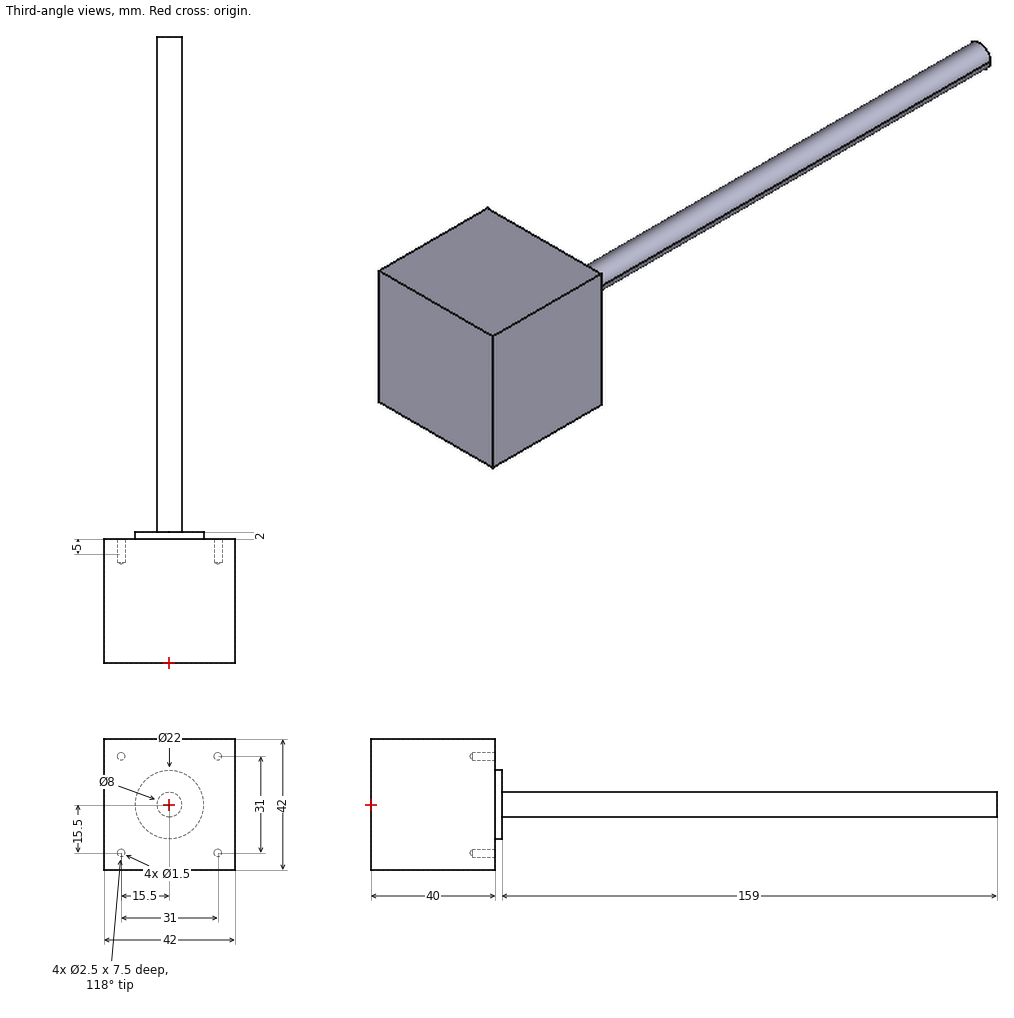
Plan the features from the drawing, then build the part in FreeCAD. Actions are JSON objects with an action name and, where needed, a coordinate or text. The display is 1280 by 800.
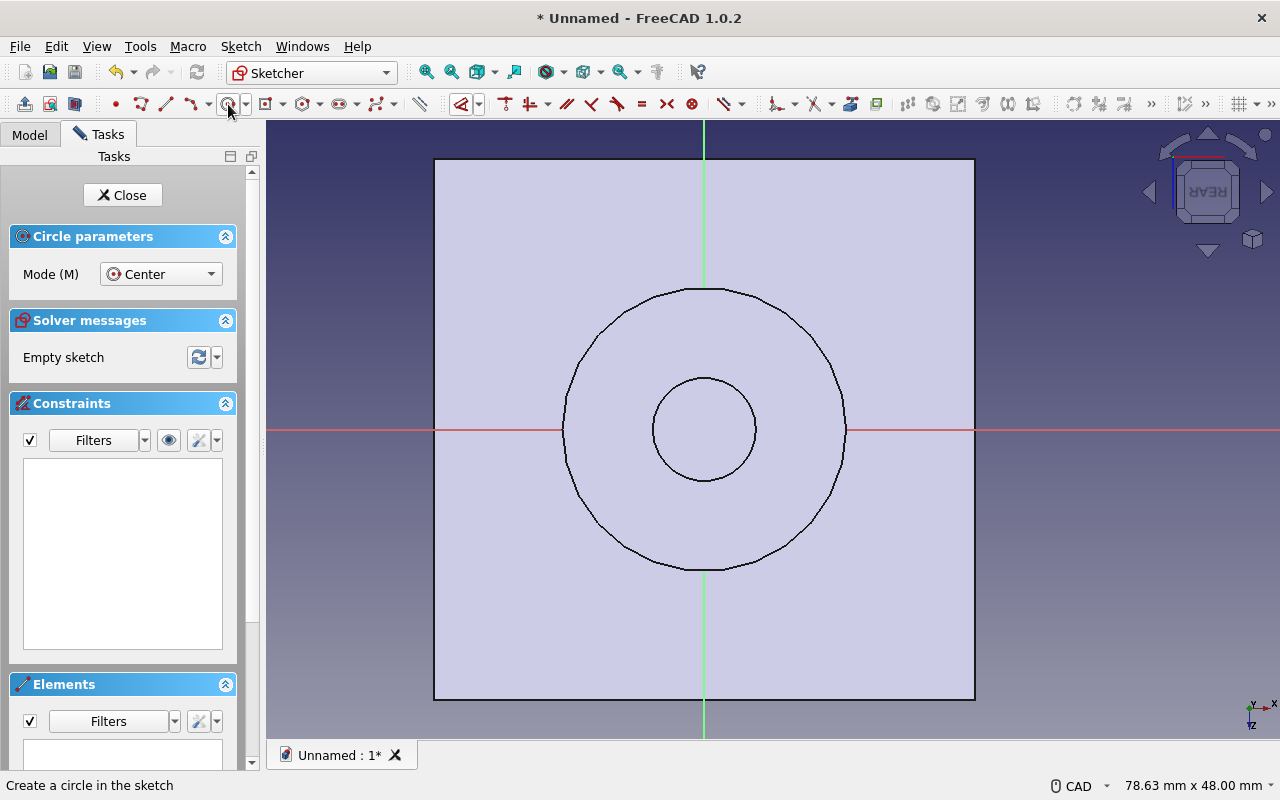
{"action": "scroll", "coordinate": [504, 230], "scroll_direction": "up", "scroll_amount": 5}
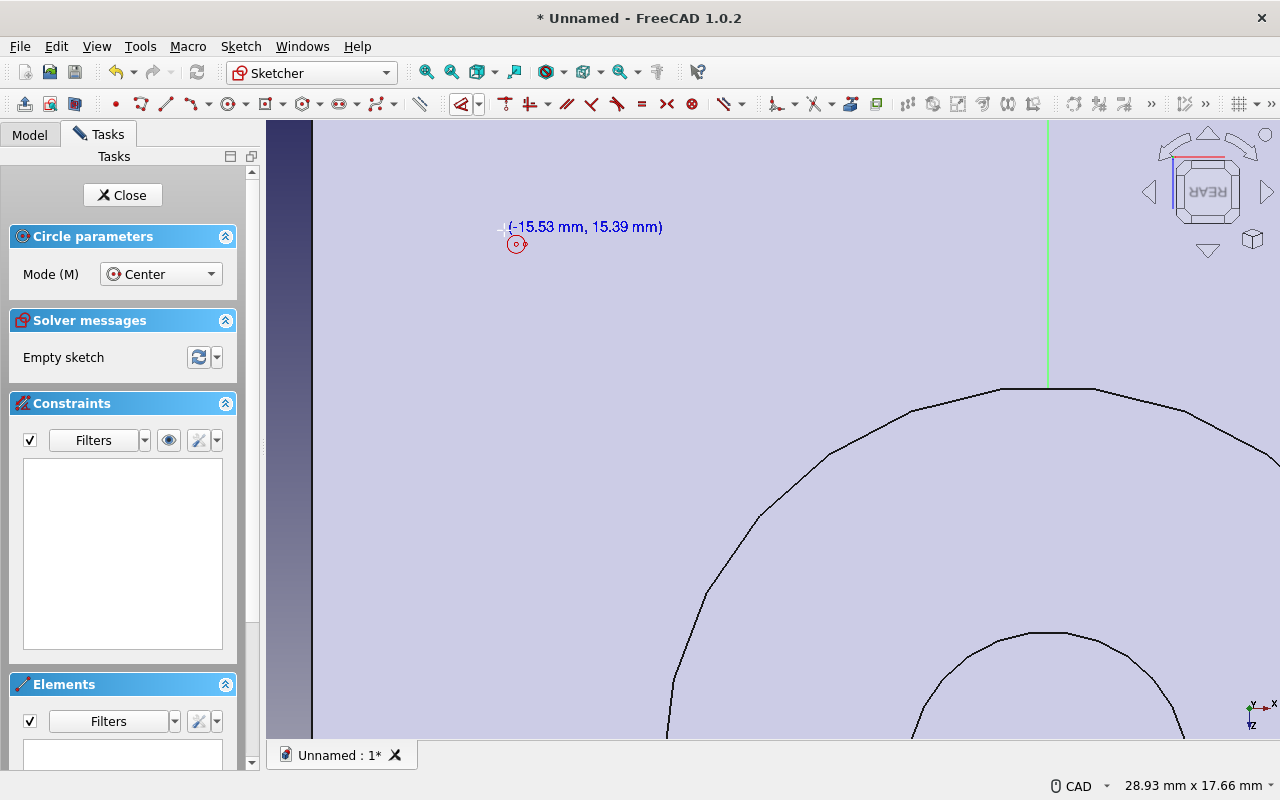
{"action": "left_click", "coordinate": [505, 229]}
{"action": "left_click", "coordinate": [523, 210]}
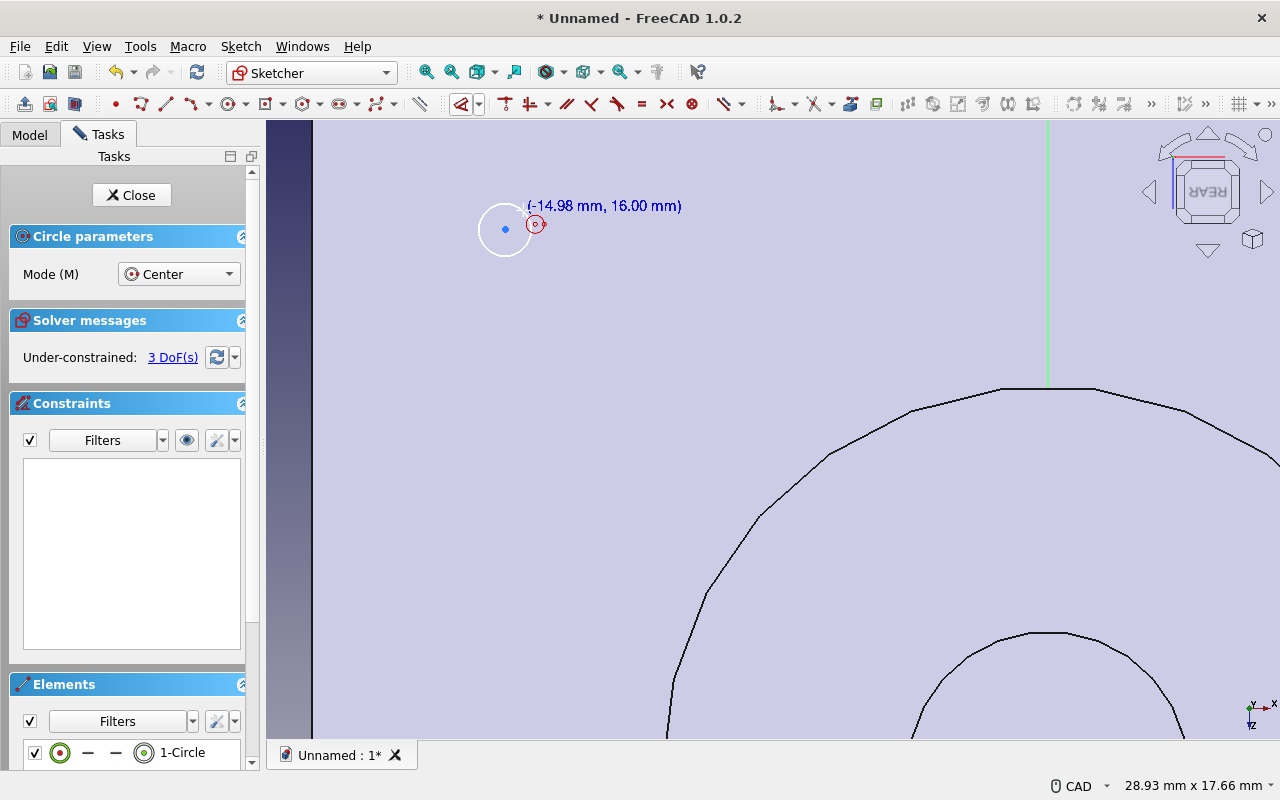
{"action": "scroll", "coordinate": [505, 230], "scroll_direction": "down", "scroll_amount": 5}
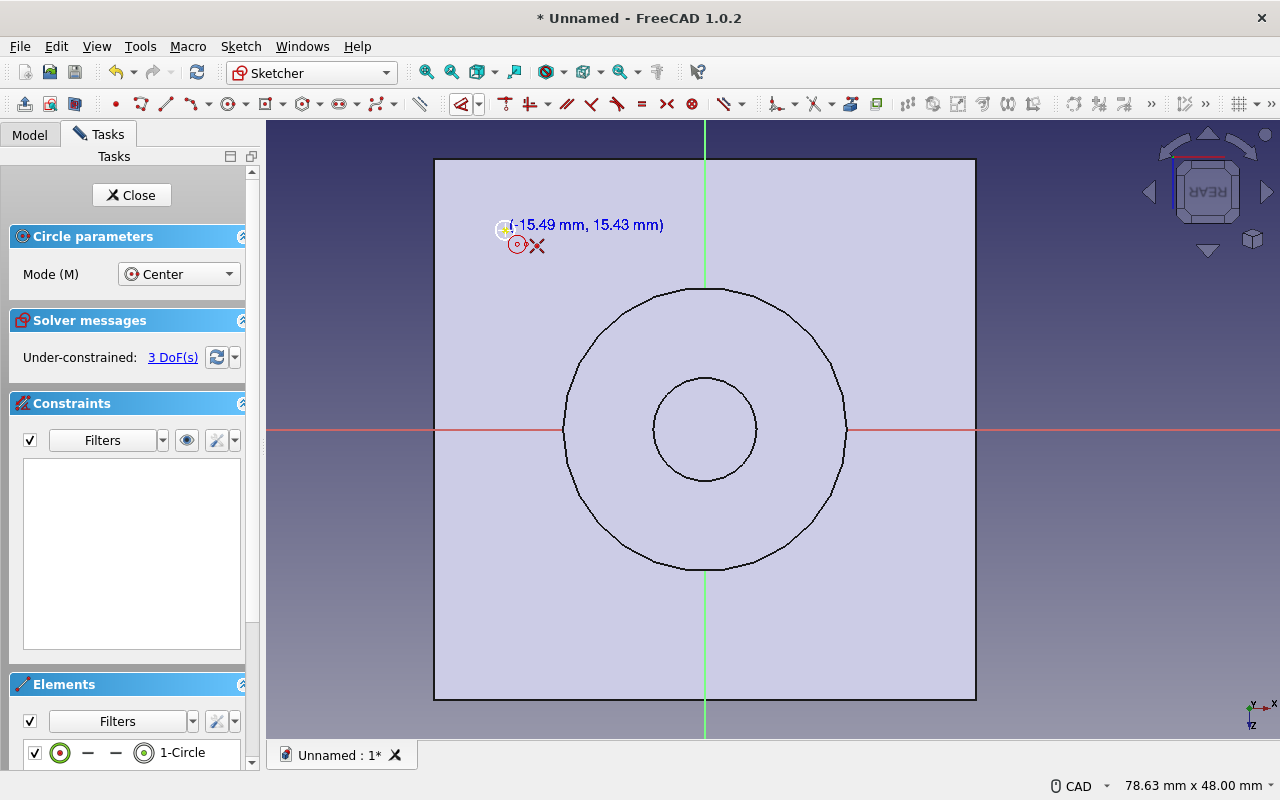
{"action": "scroll", "coordinate": [905, 230], "scroll_direction": "up", "scroll_amount": 5}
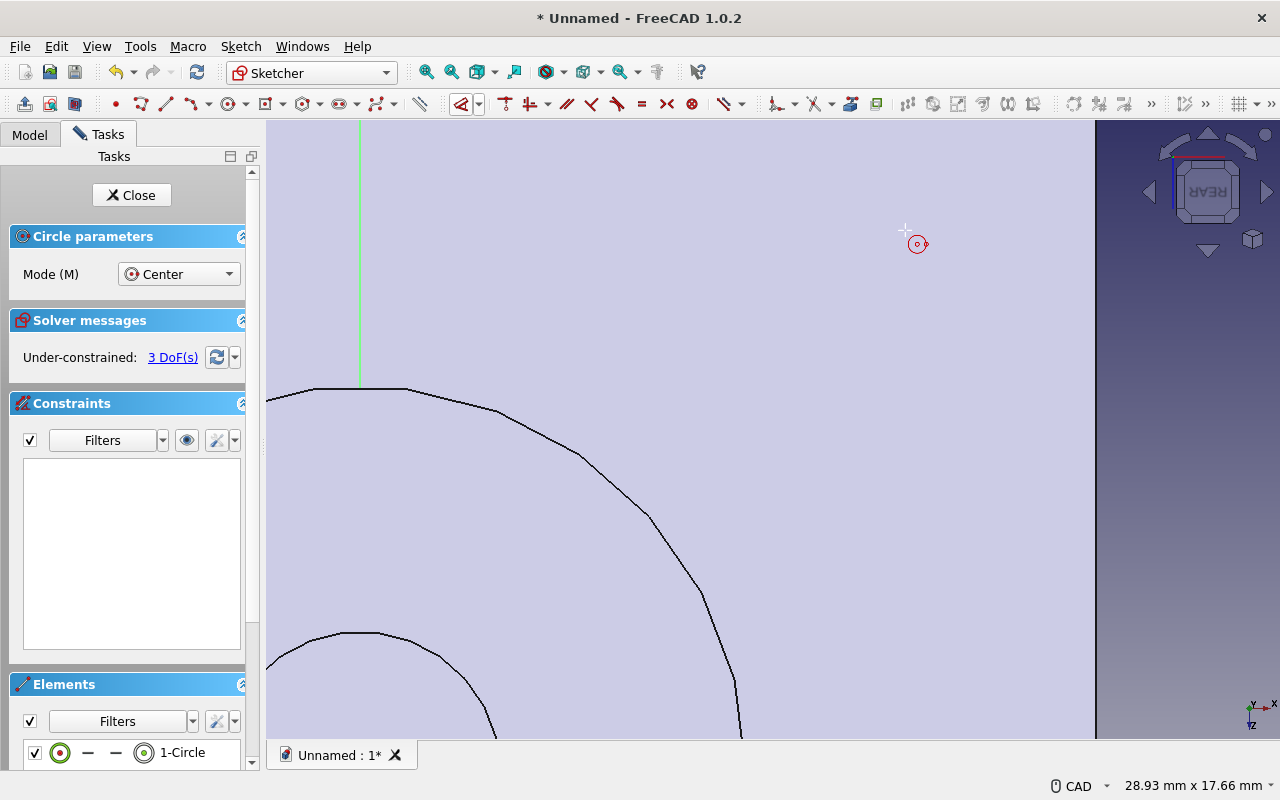
{"action": "left_click", "coordinate": [903, 229]}
{"action": "left_click", "coordinate": [922, 210]}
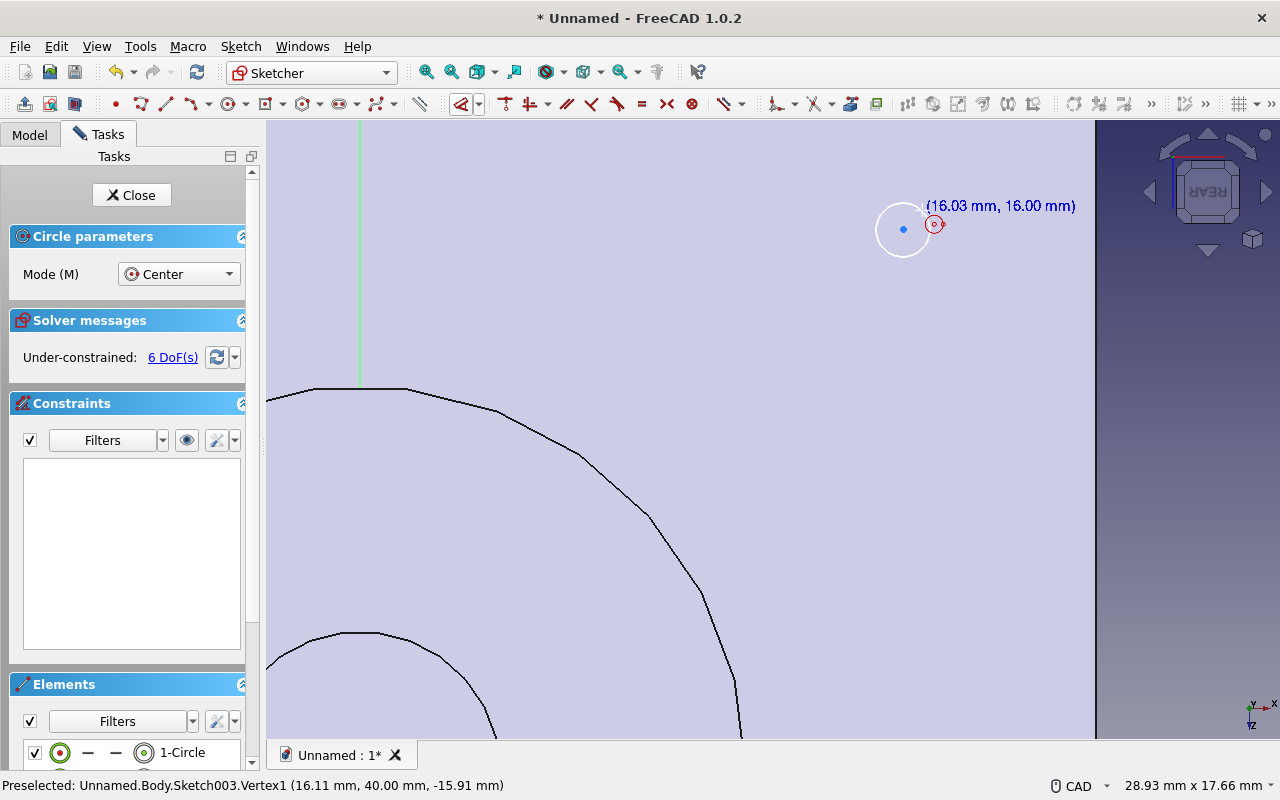
{"action": "scroll", "coordinate": [905, 230], "scroll_direction": "down", "scroll_amount": 5}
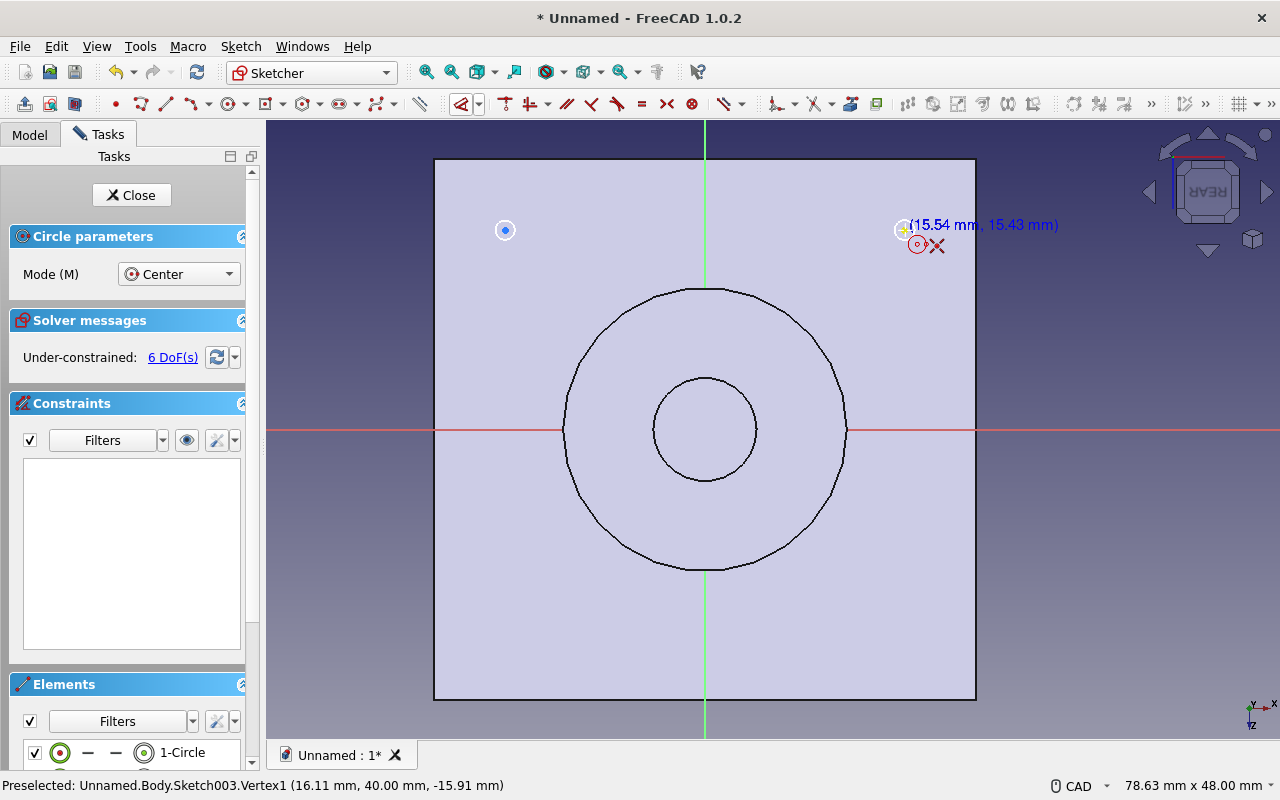
{"action": "scroll", "coordinate": [905, 629], "scroll_direction": "up", "scroll_amount": 5}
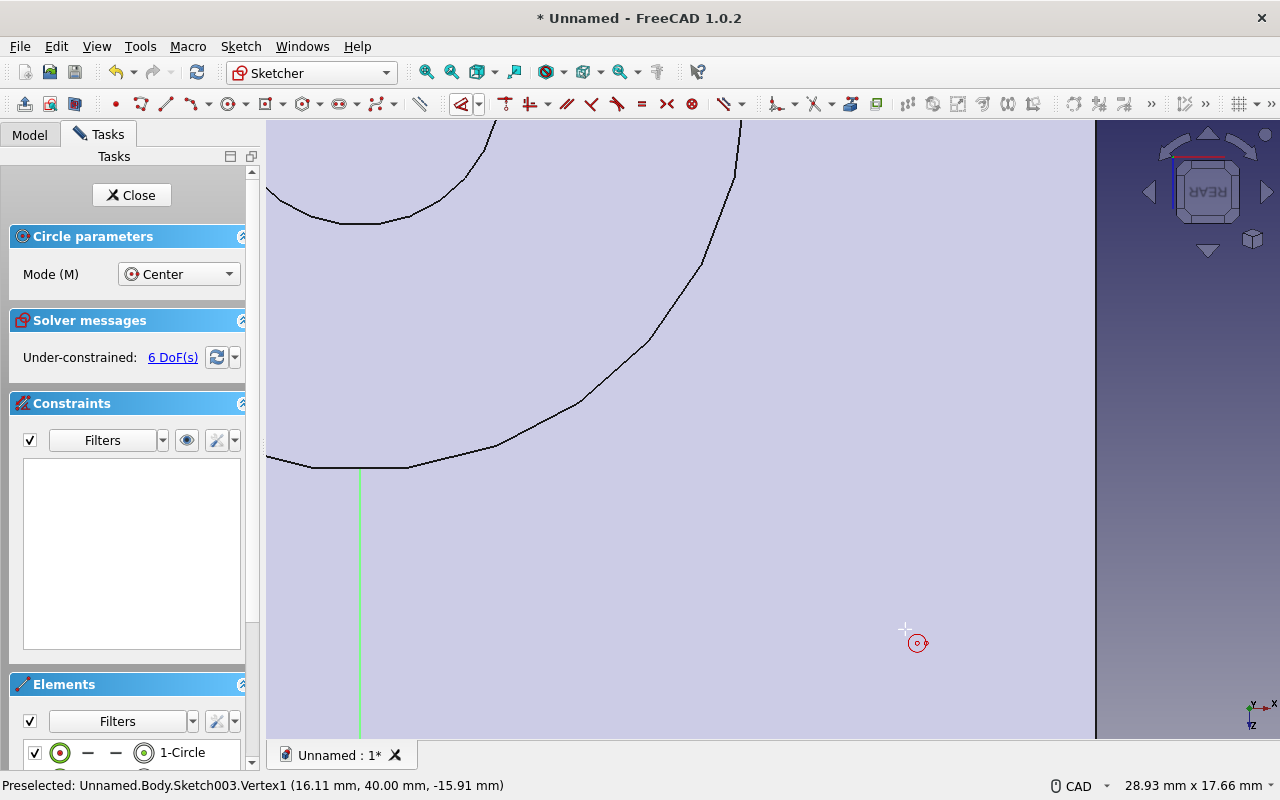
{"action": "left_click", "coordinate": [903, 629]}
{"action": "left_click", "coordinate": [922, 610]}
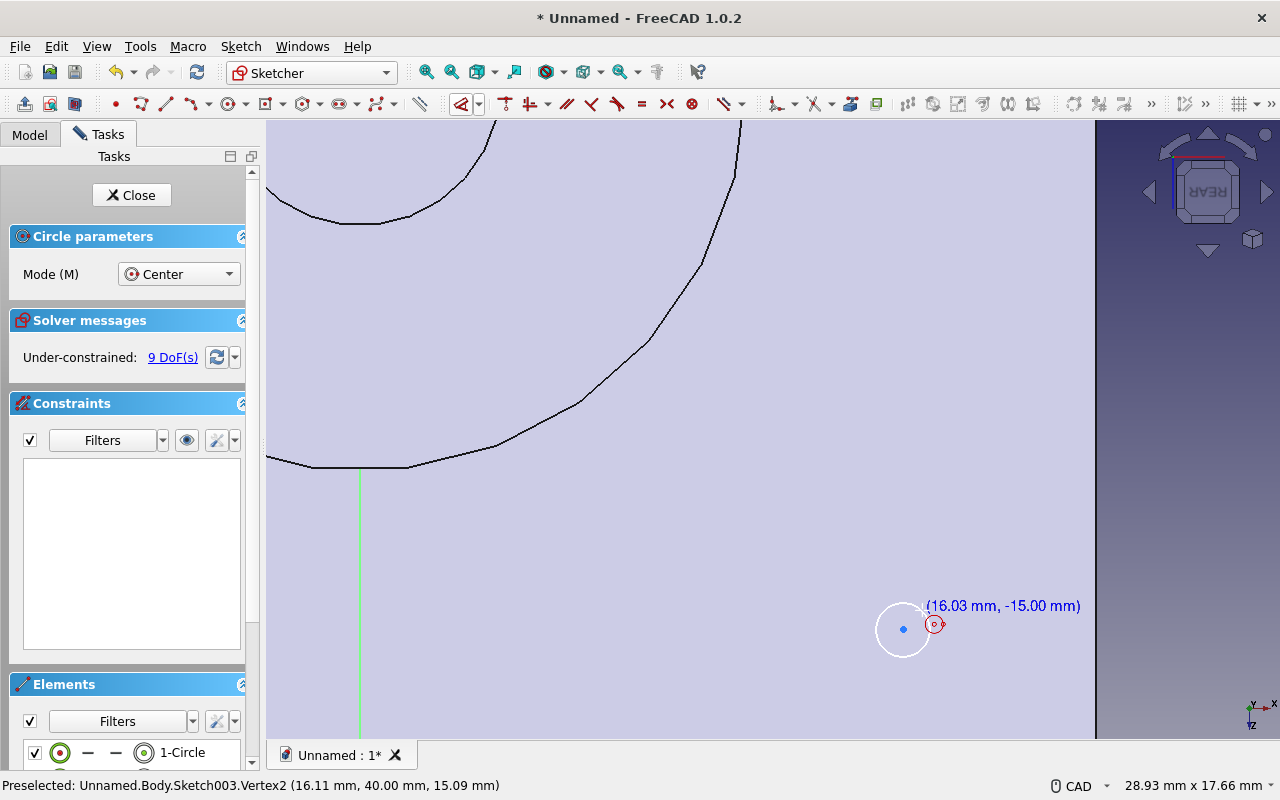
{"action": "scroll", "coordinate": [905, 630], "scroll_direction": "down", "scroll_amount": 5}